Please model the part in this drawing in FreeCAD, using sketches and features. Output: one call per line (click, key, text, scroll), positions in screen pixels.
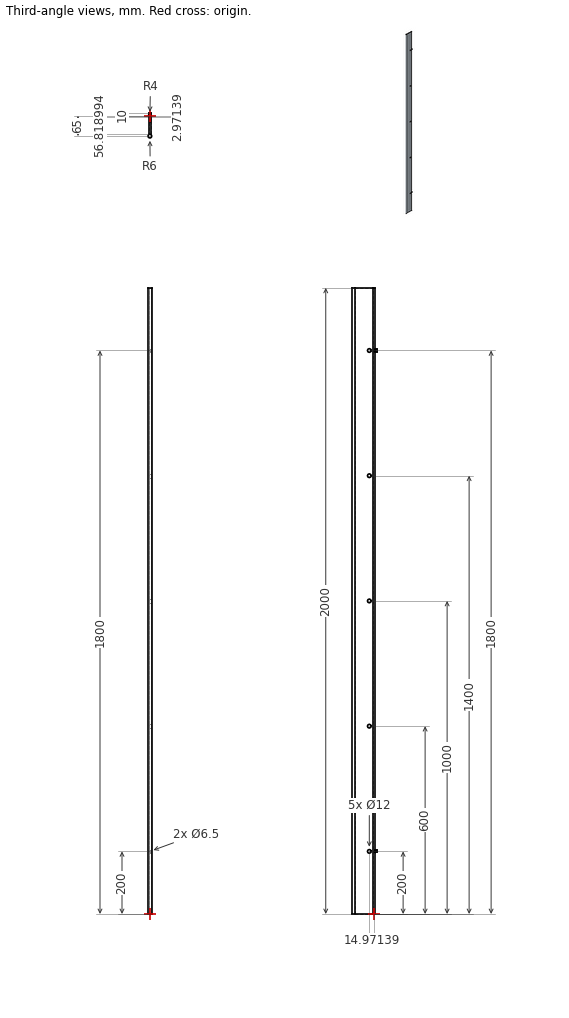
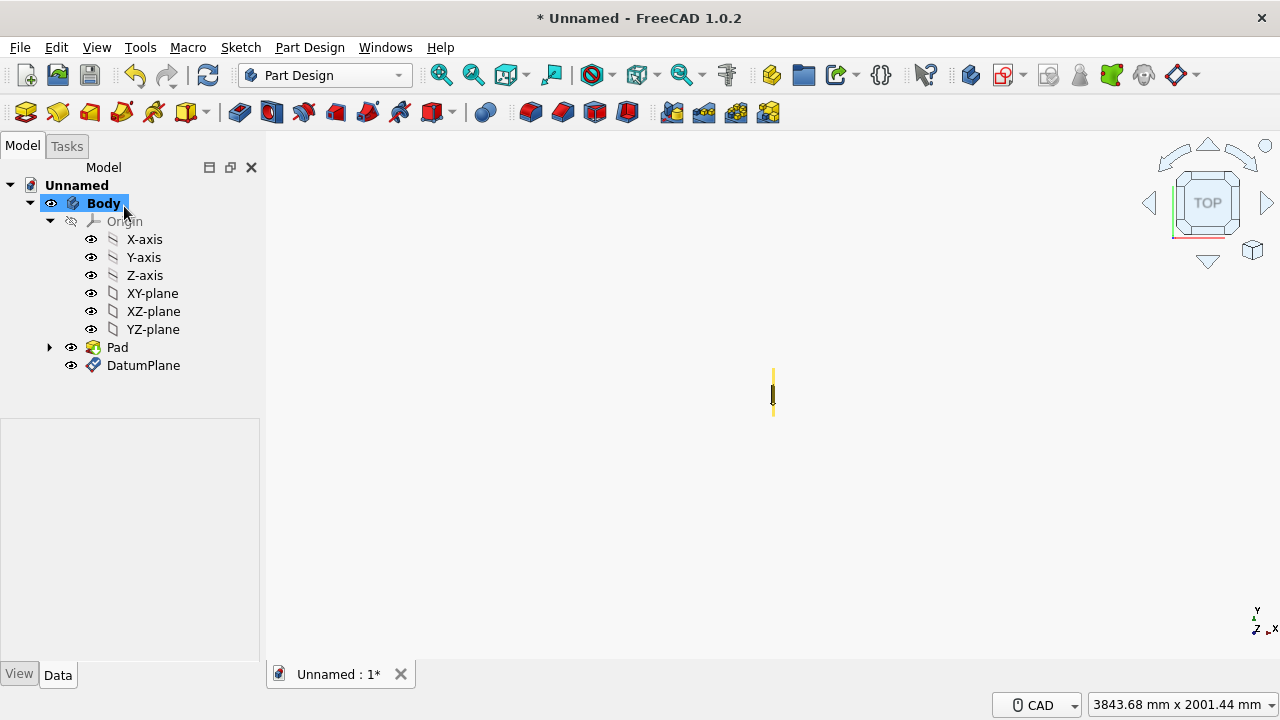
click(116, 365)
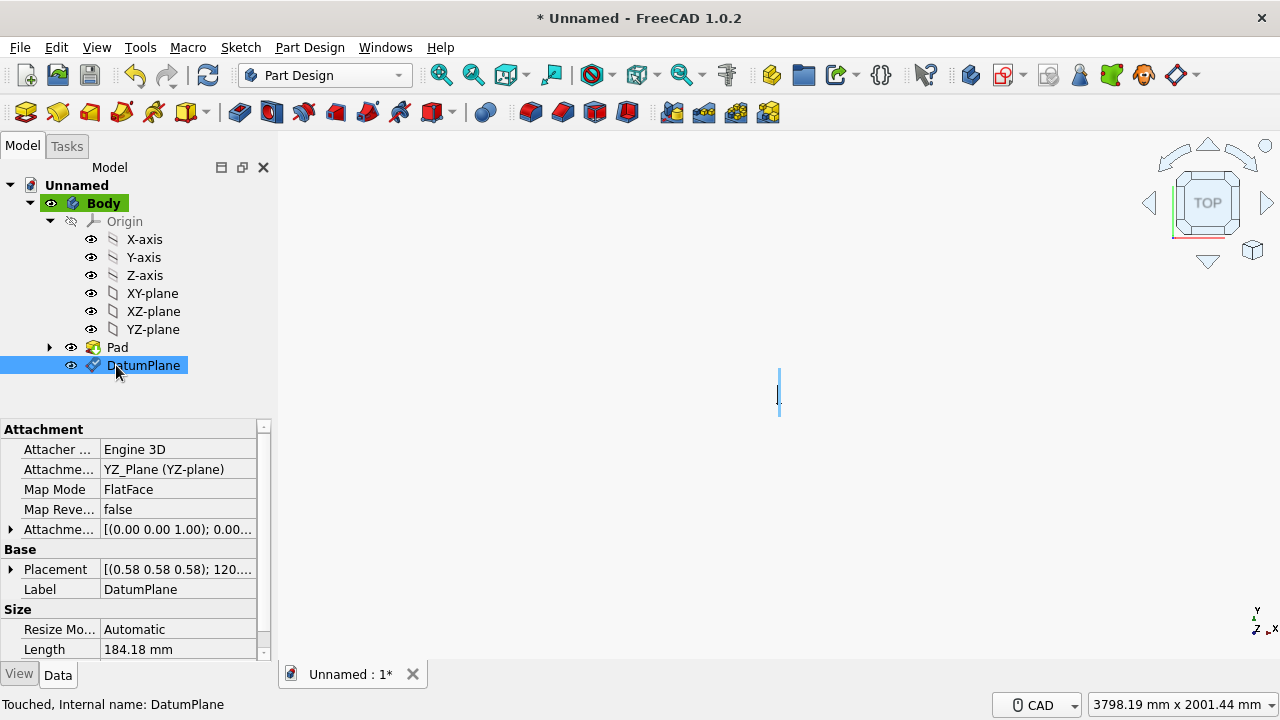
click(1004, 76)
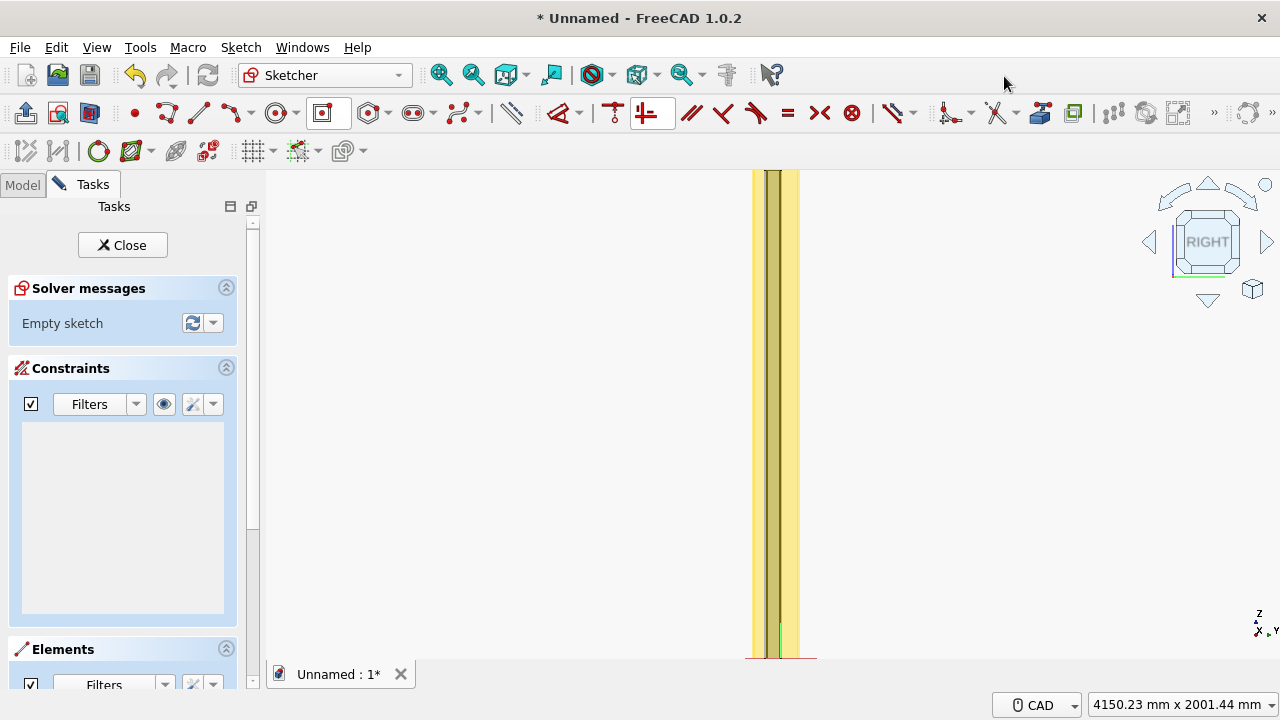
key(q)
key(s)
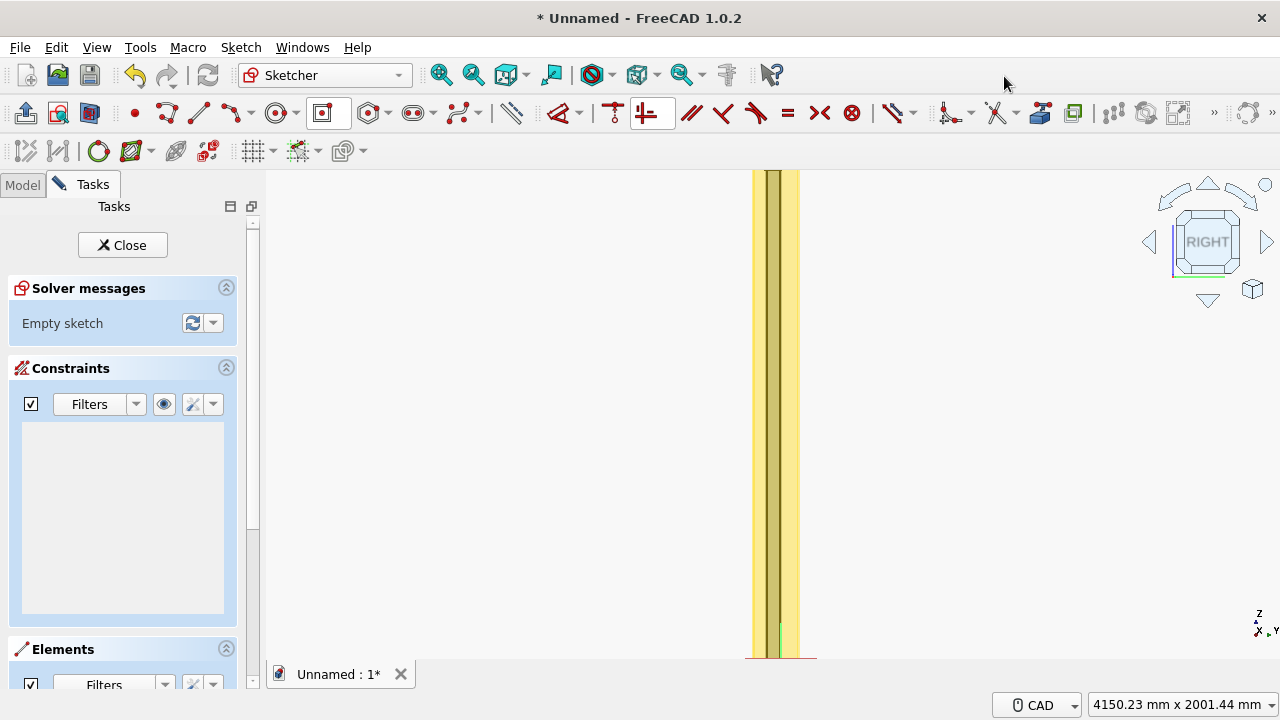
scroll(554, 366, down, 2)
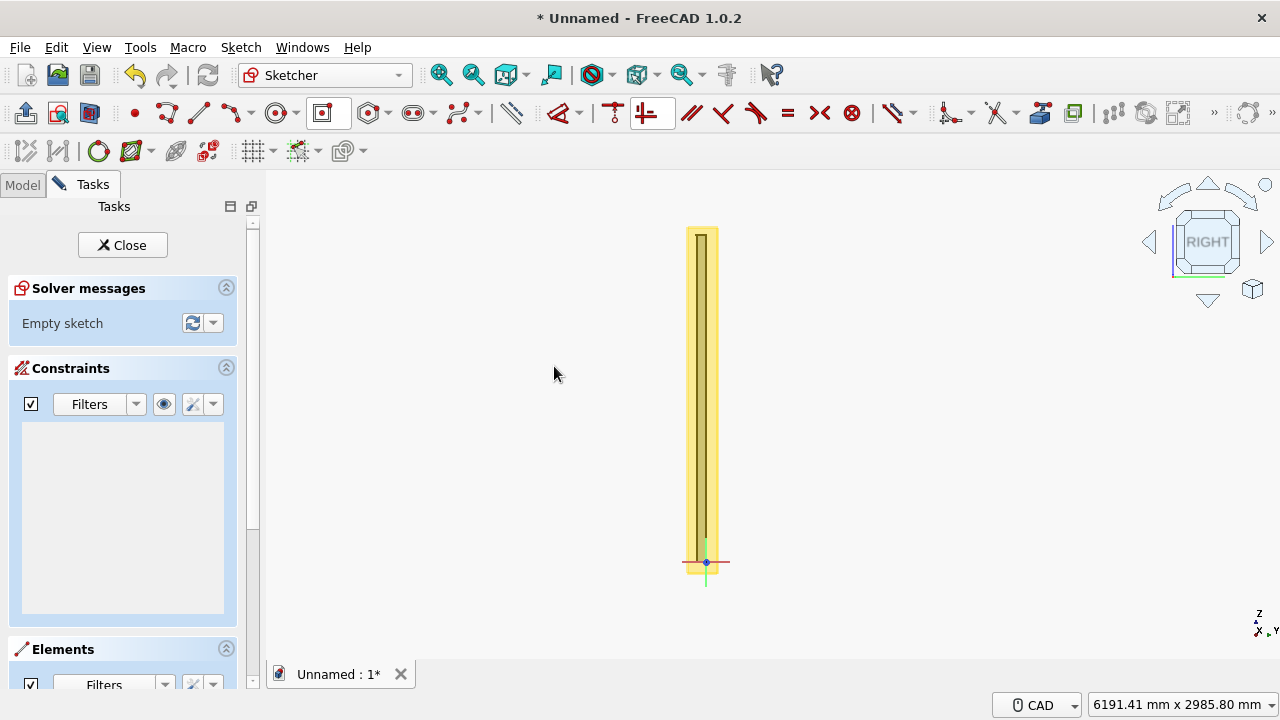
click(276, 114)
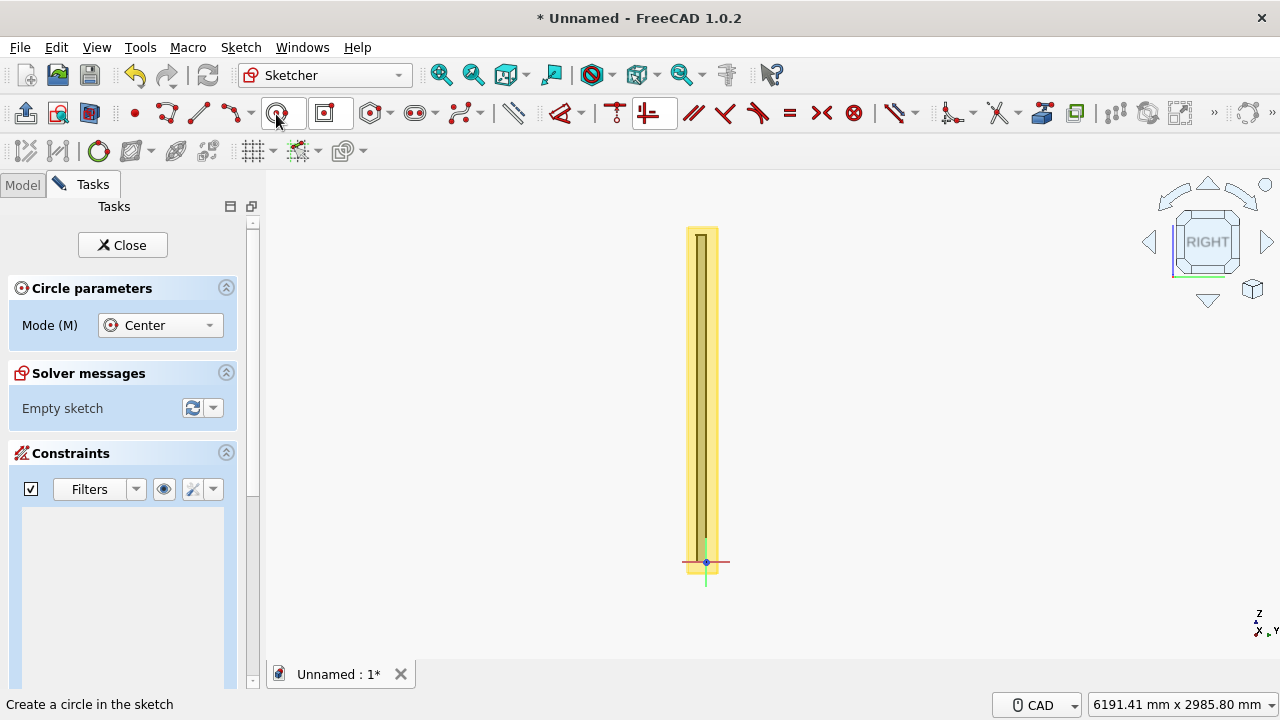
scroll(704, 530, up, 16)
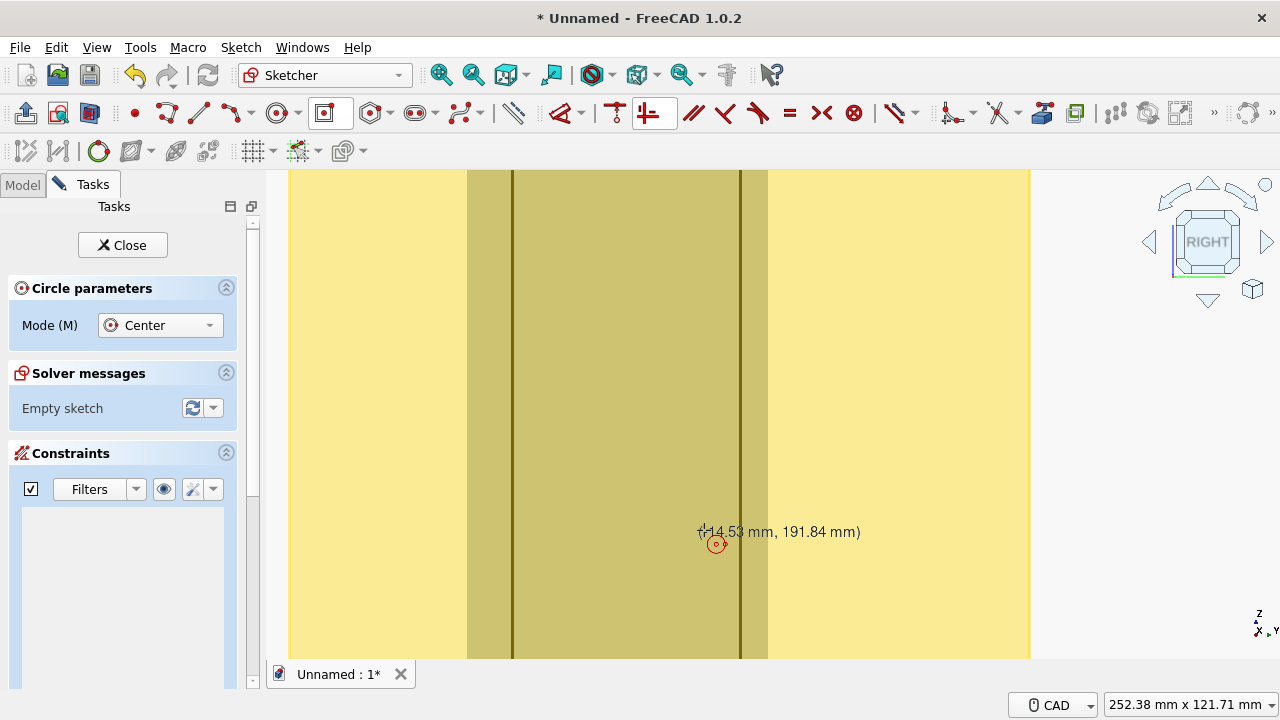
scroll(704, 558, down, 15)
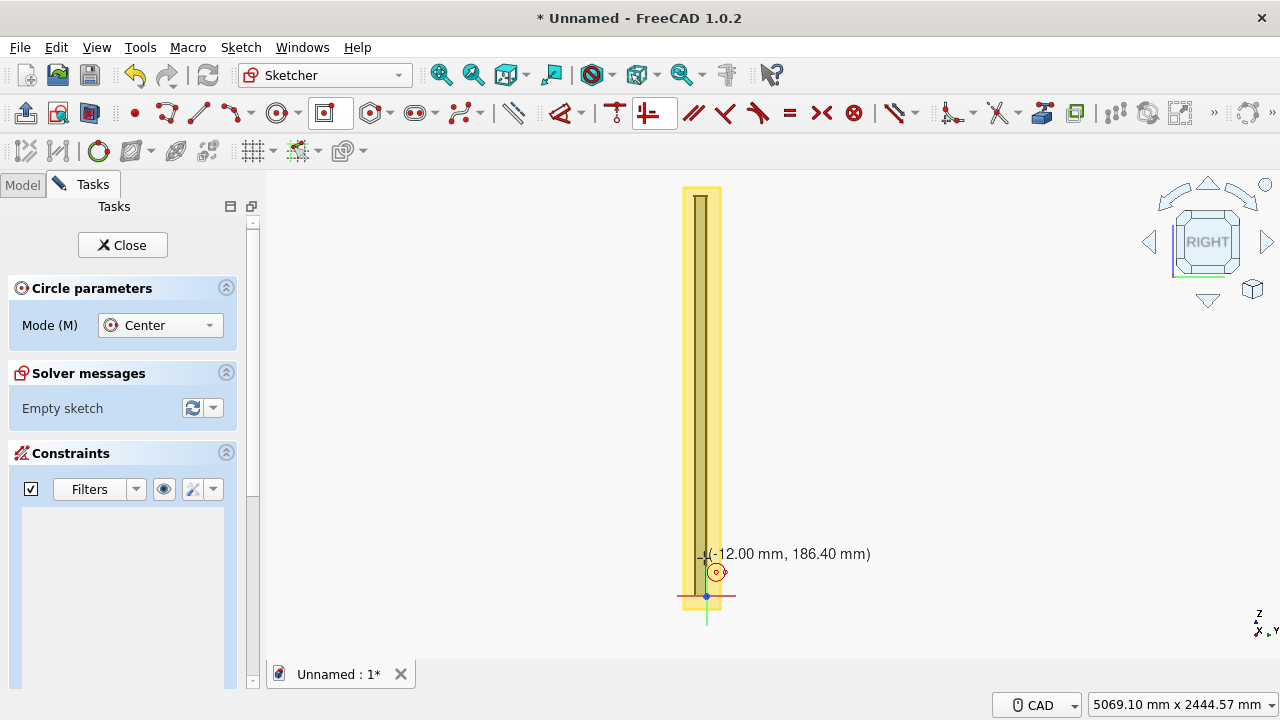
scroll(704, 556, up, 9)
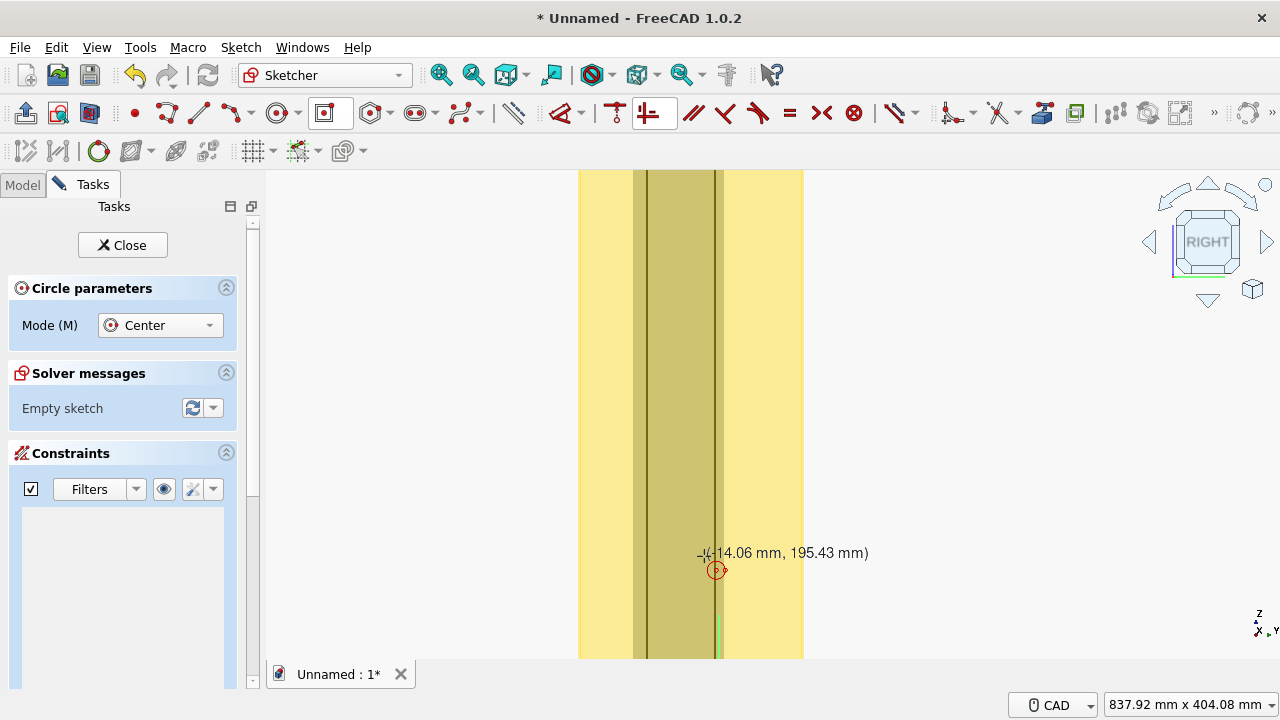
click(701, 553)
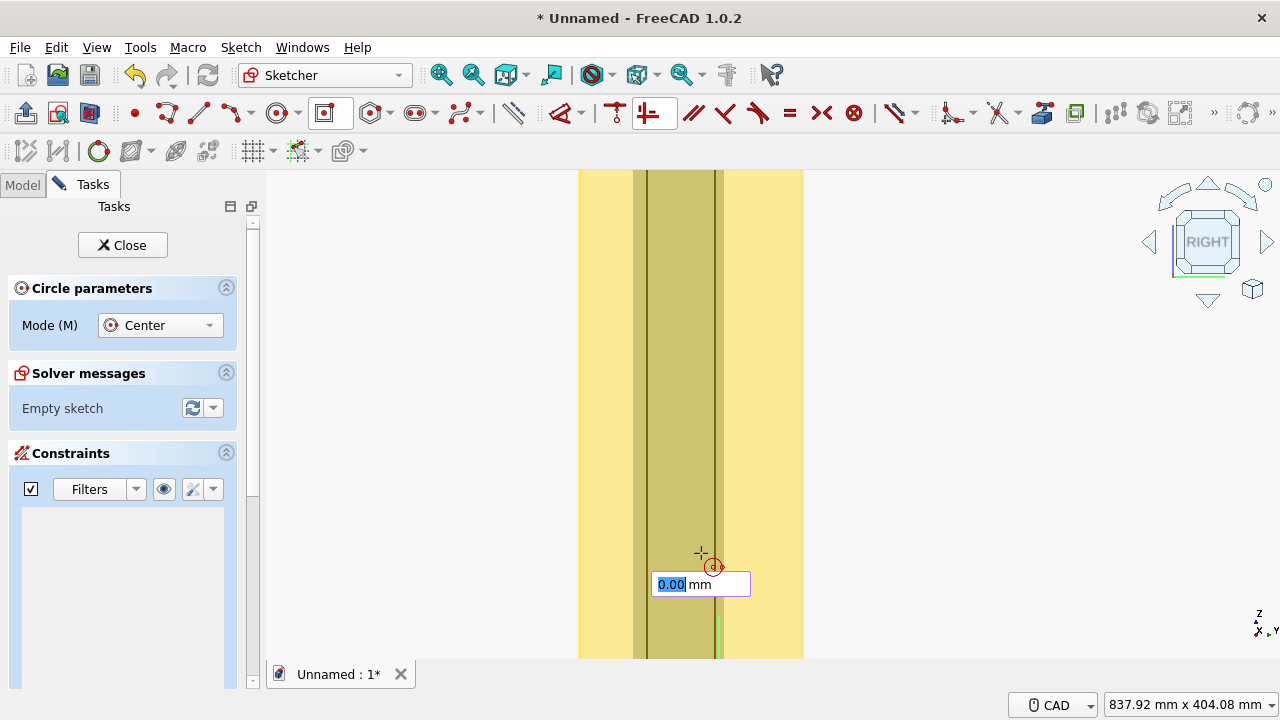
scroll(696, 547, up, 4)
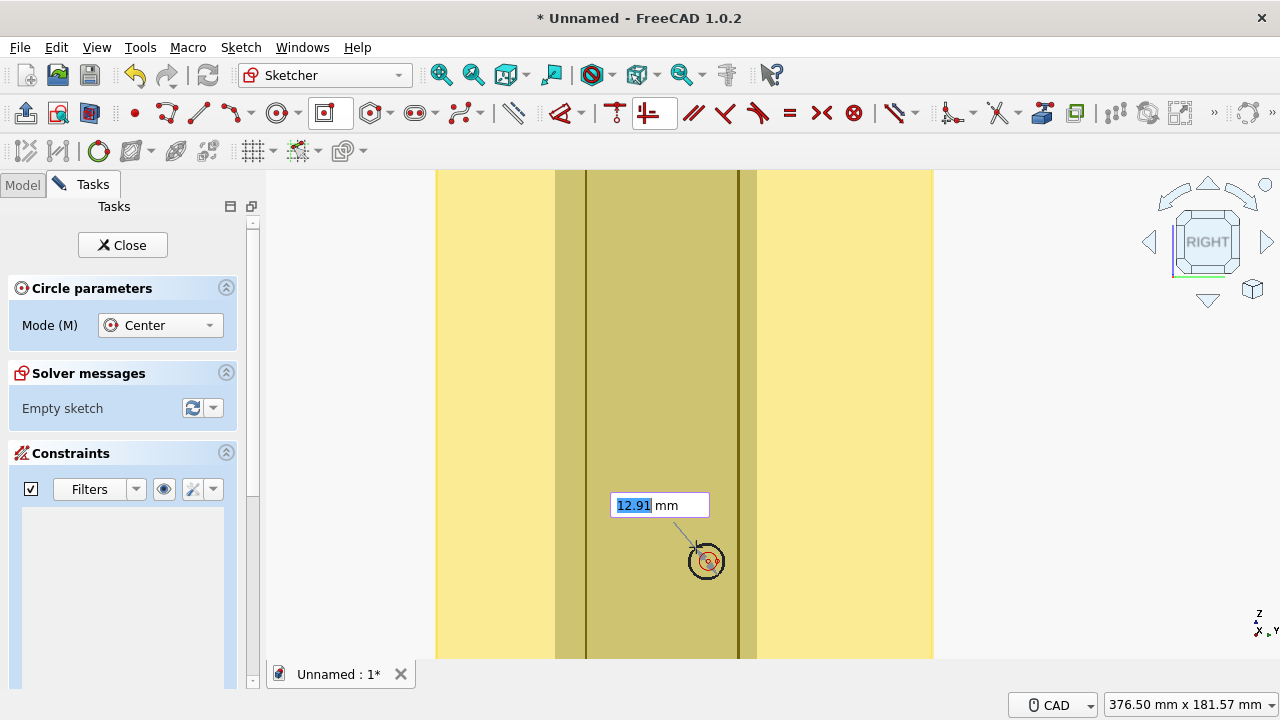
click(695, 547)